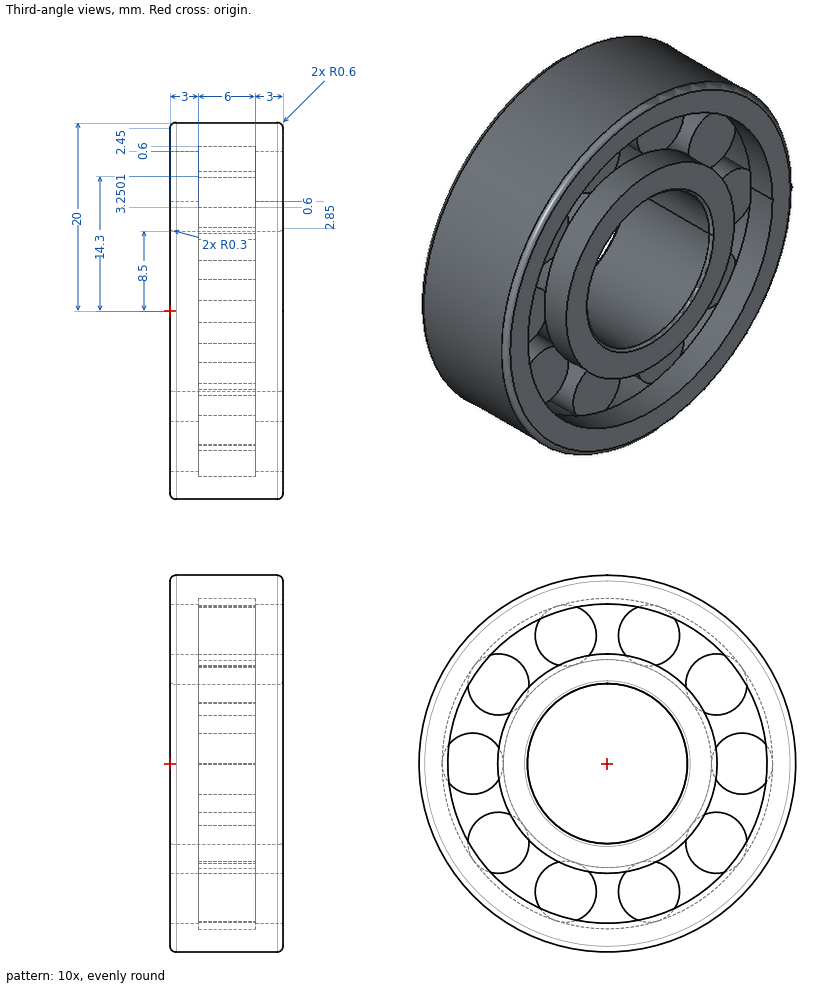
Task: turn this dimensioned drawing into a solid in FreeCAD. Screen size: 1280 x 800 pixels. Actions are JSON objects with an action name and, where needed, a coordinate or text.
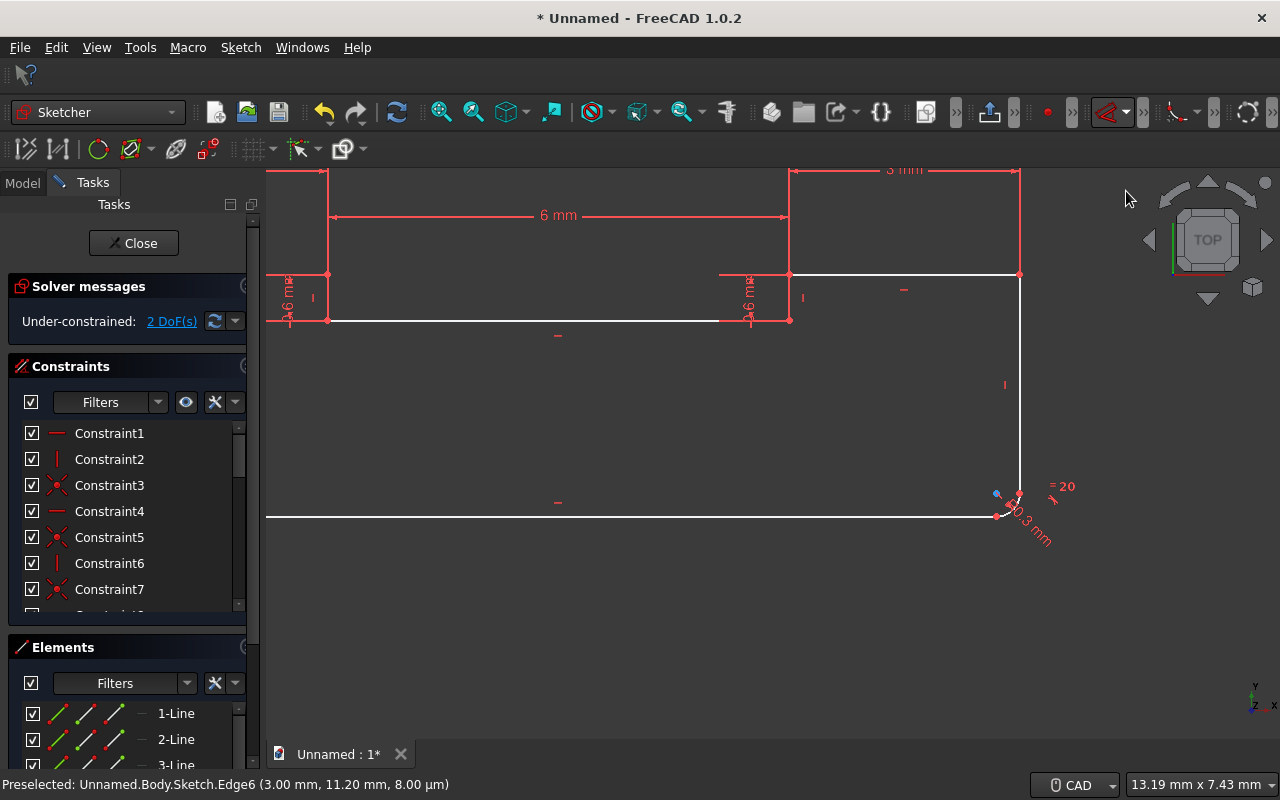
{"action": "left_click", "coordinate": [1020, 428]}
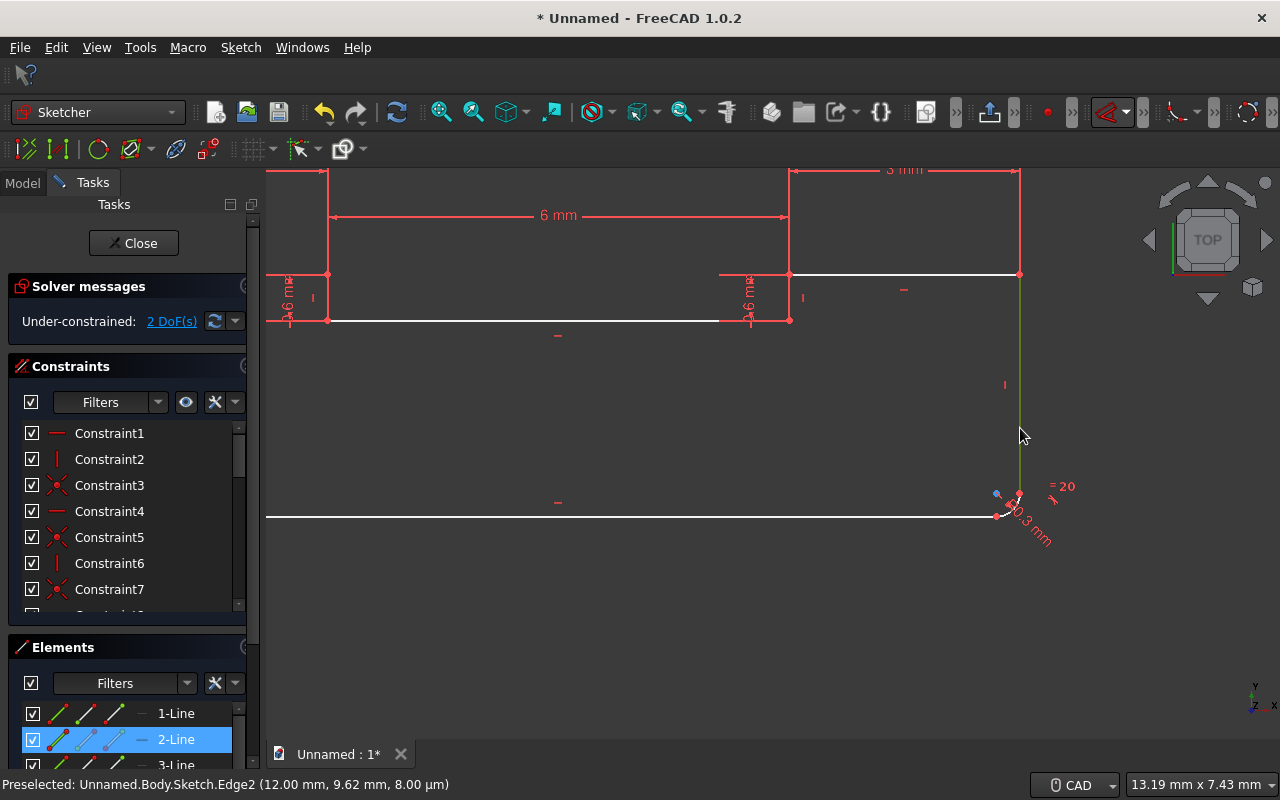
{"action": "left_click", "coordinate": [1128, 112]}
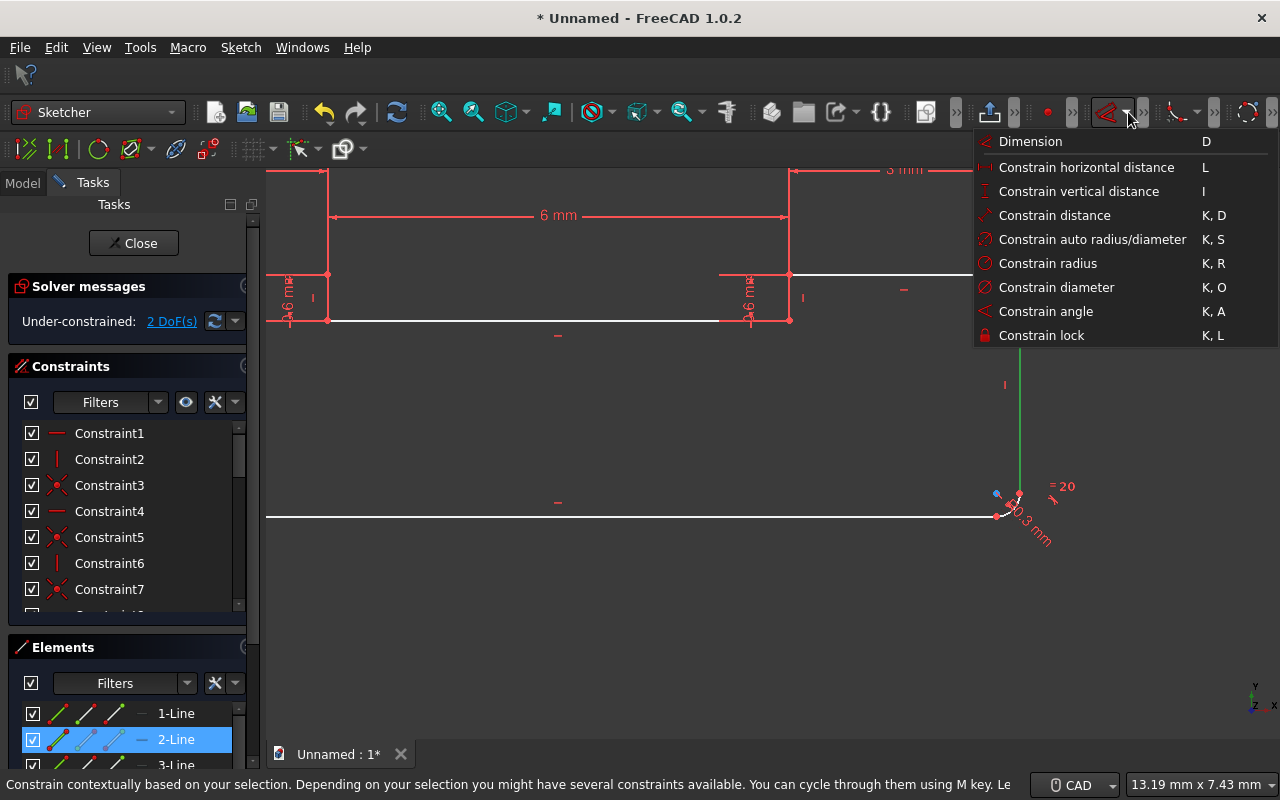
{"action": "left_click", "coordinate": [1126, 191]}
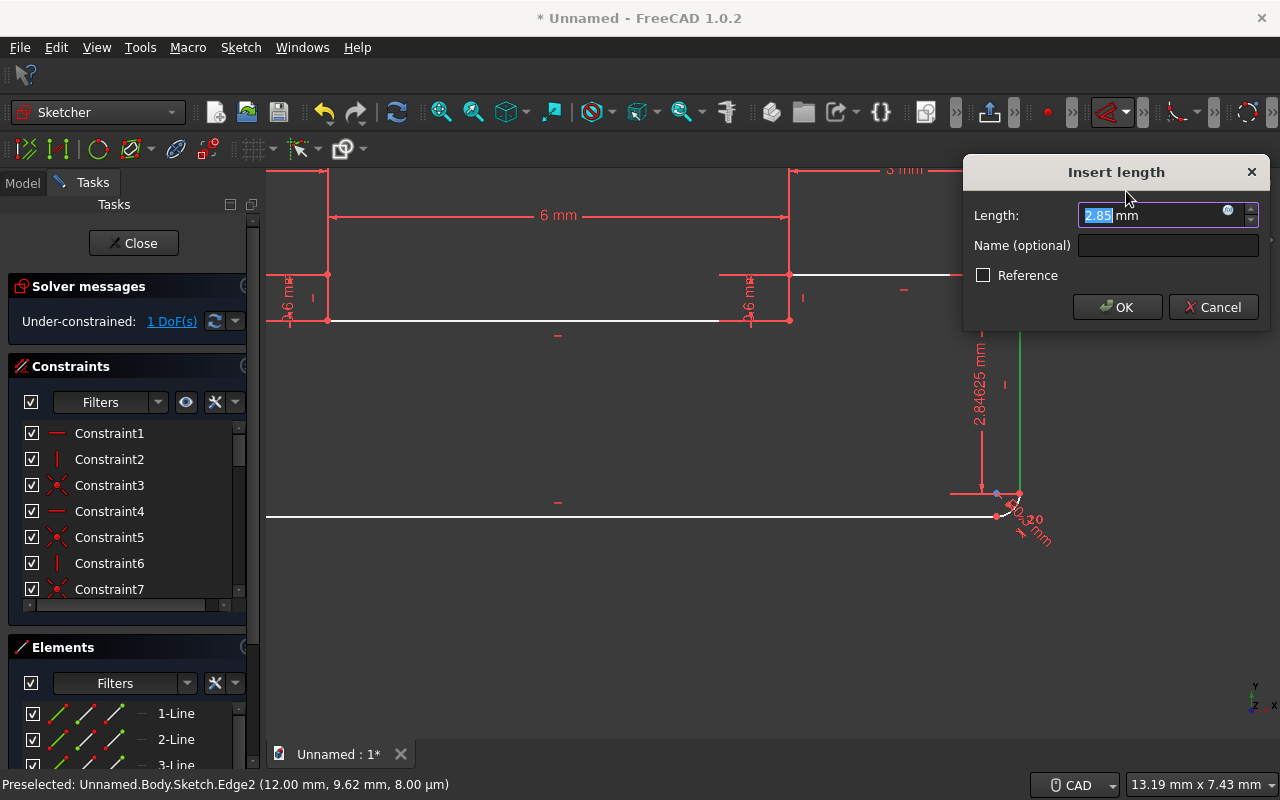
{"action": "type", "text": "2.85"}
{"action": "key", "text": "Return"}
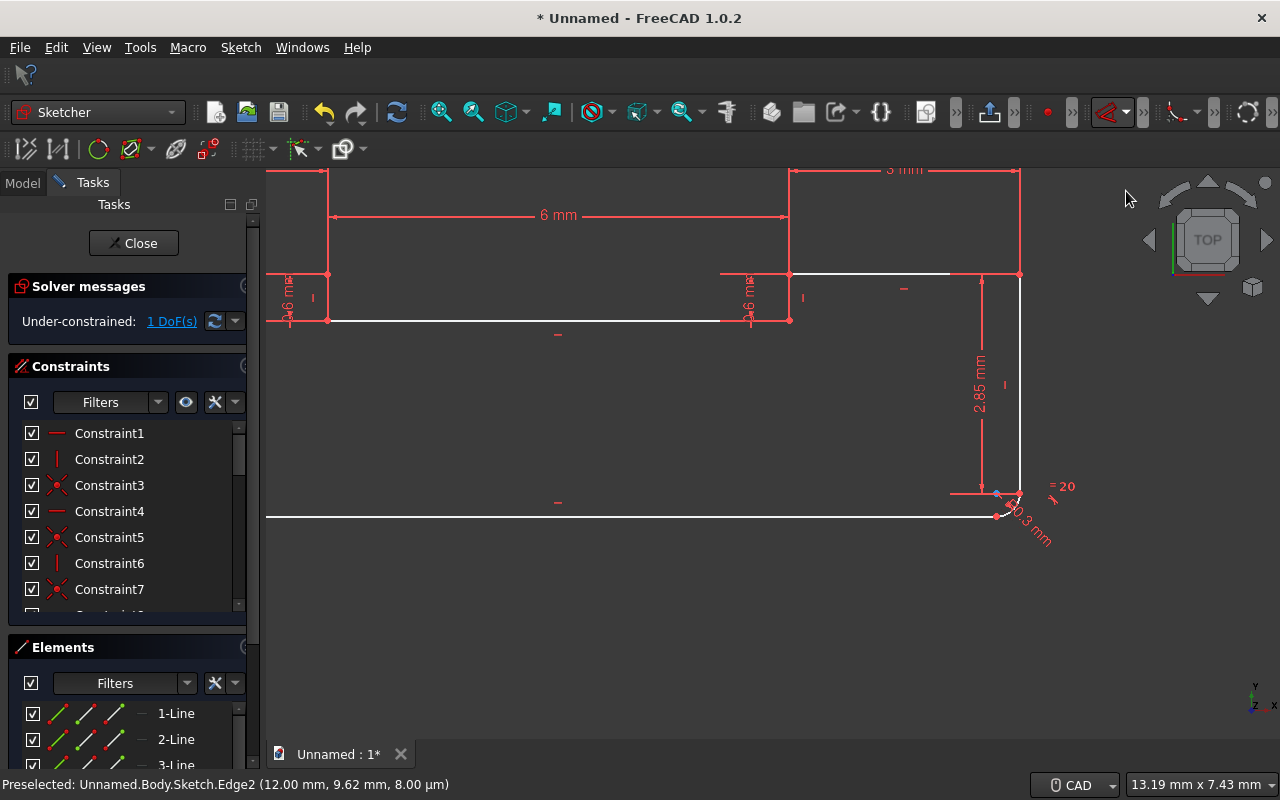
{"action": "scroll", "coordinate": [789, 298], "scroll_direction": "down", "scroll_amount": 5}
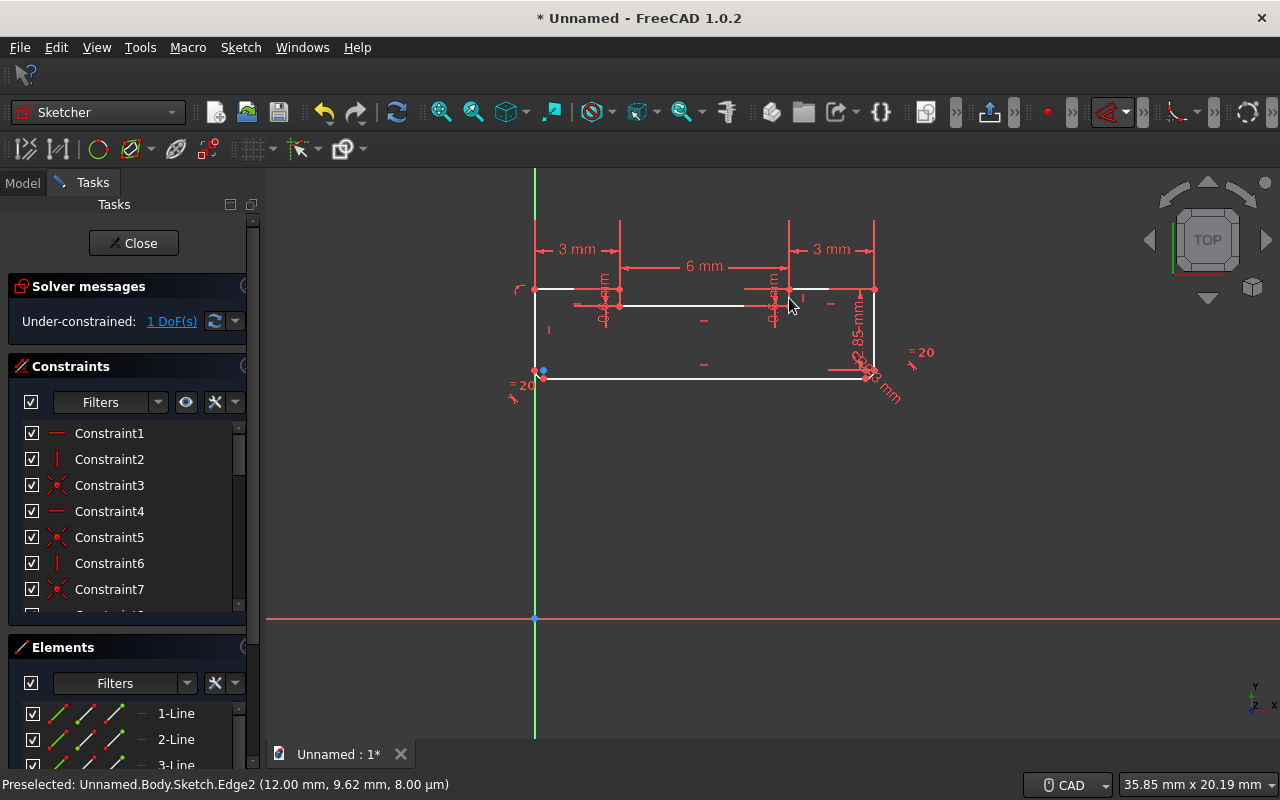
{"action": "scroll", "coordinate": [543, 379], "scroll_direction": "up", "scroll_amount": 2}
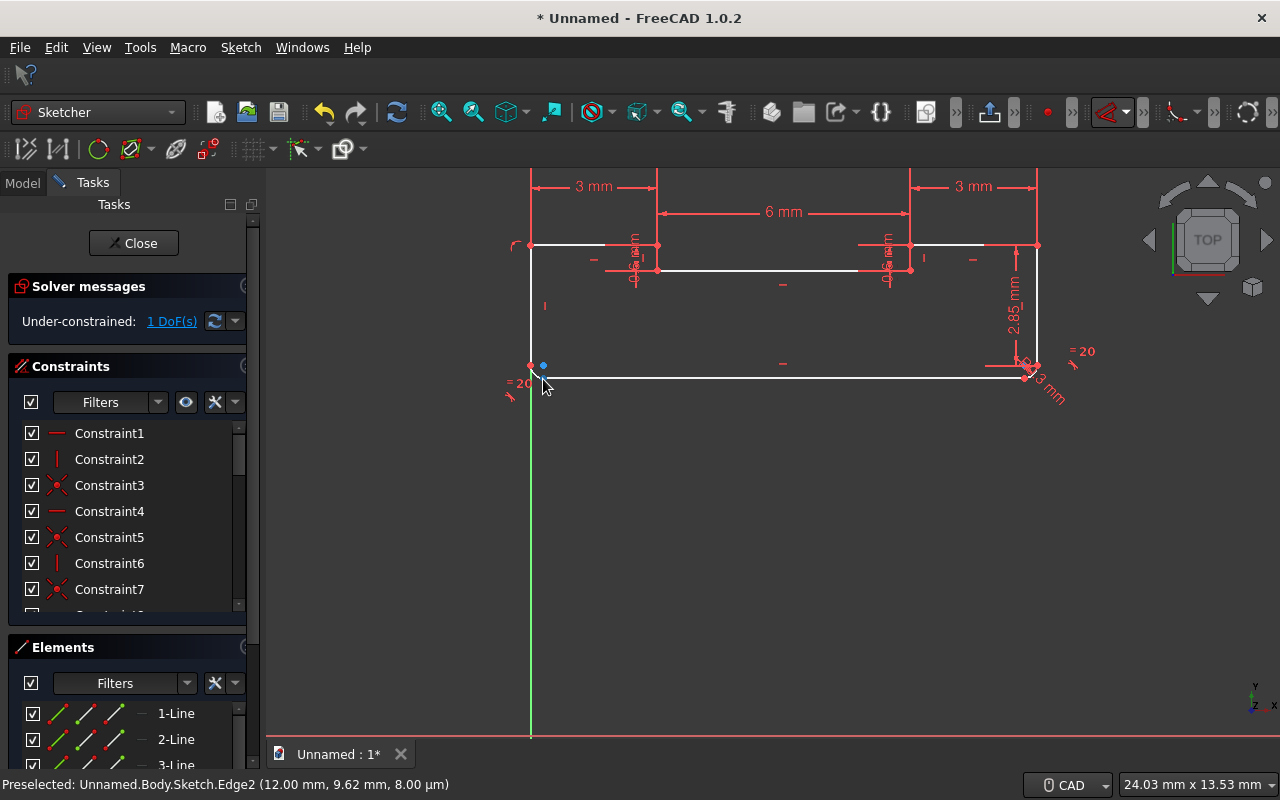
{"action": "left_click", "coordinate": [543, 378]}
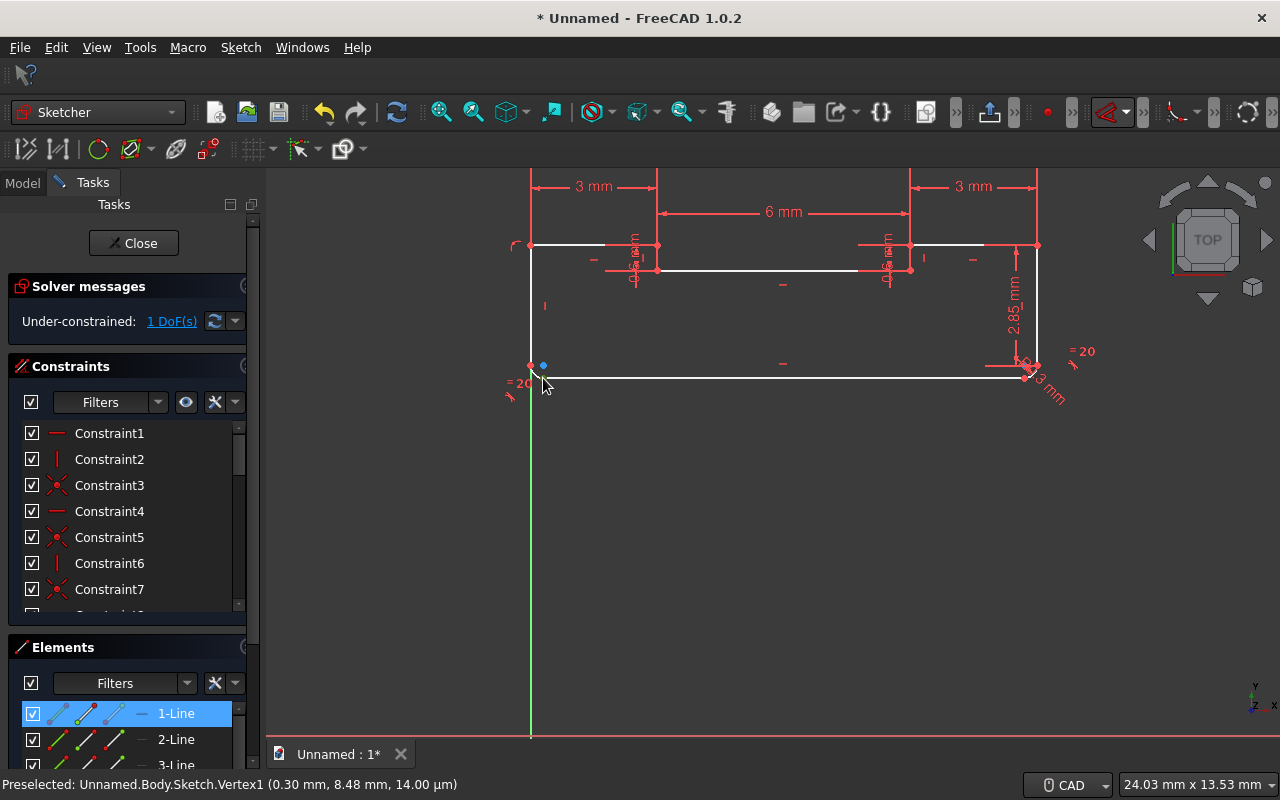
{"action": "left_click", "coordinate": [1128, 112]}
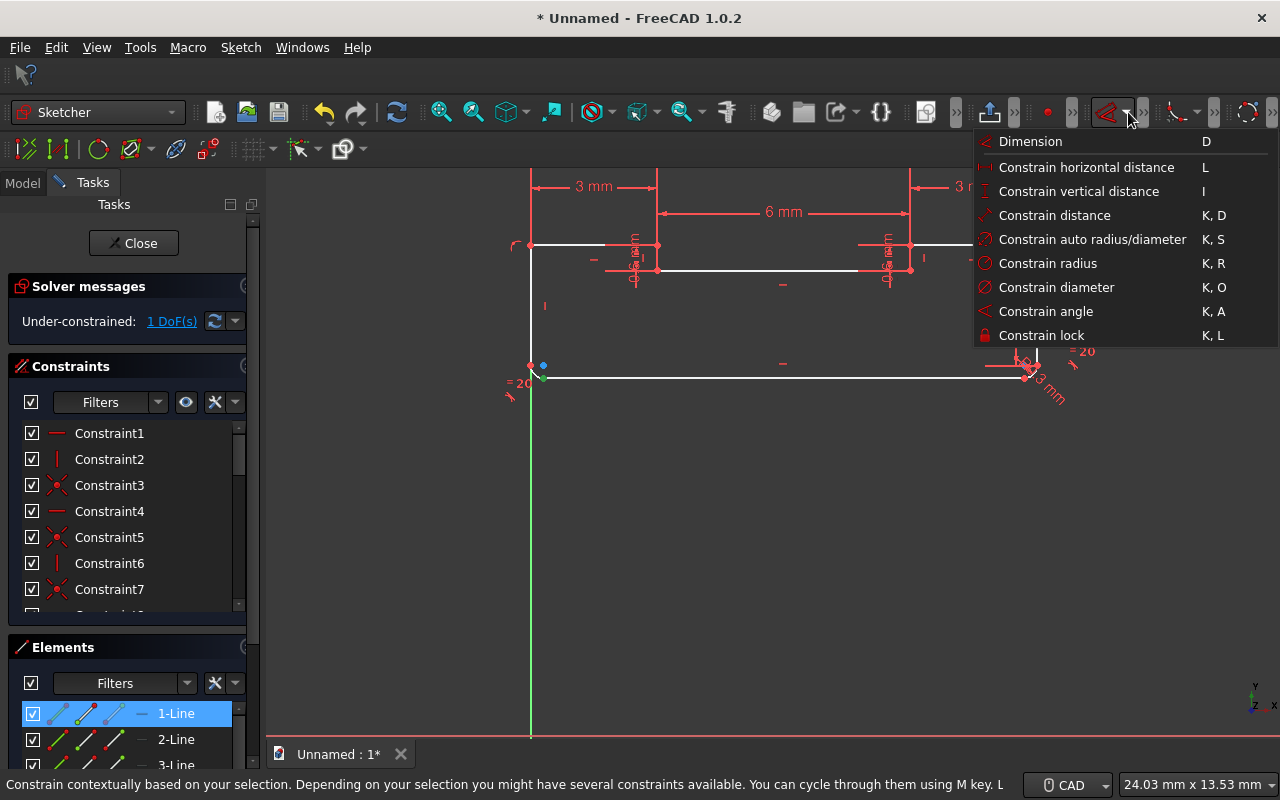
{"action": "left_click", "coordinate": [1126, 191]}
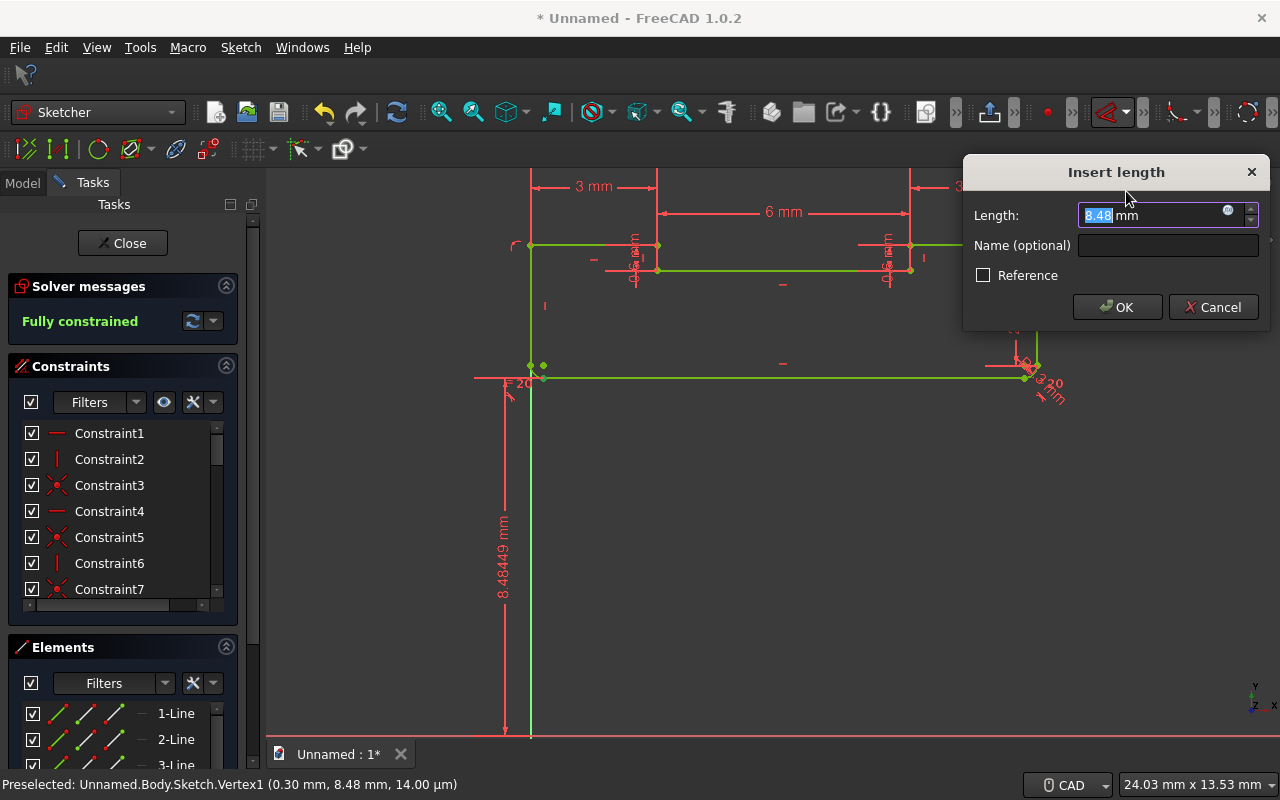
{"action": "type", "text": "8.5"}
{"action": "key", "text": "Return"}